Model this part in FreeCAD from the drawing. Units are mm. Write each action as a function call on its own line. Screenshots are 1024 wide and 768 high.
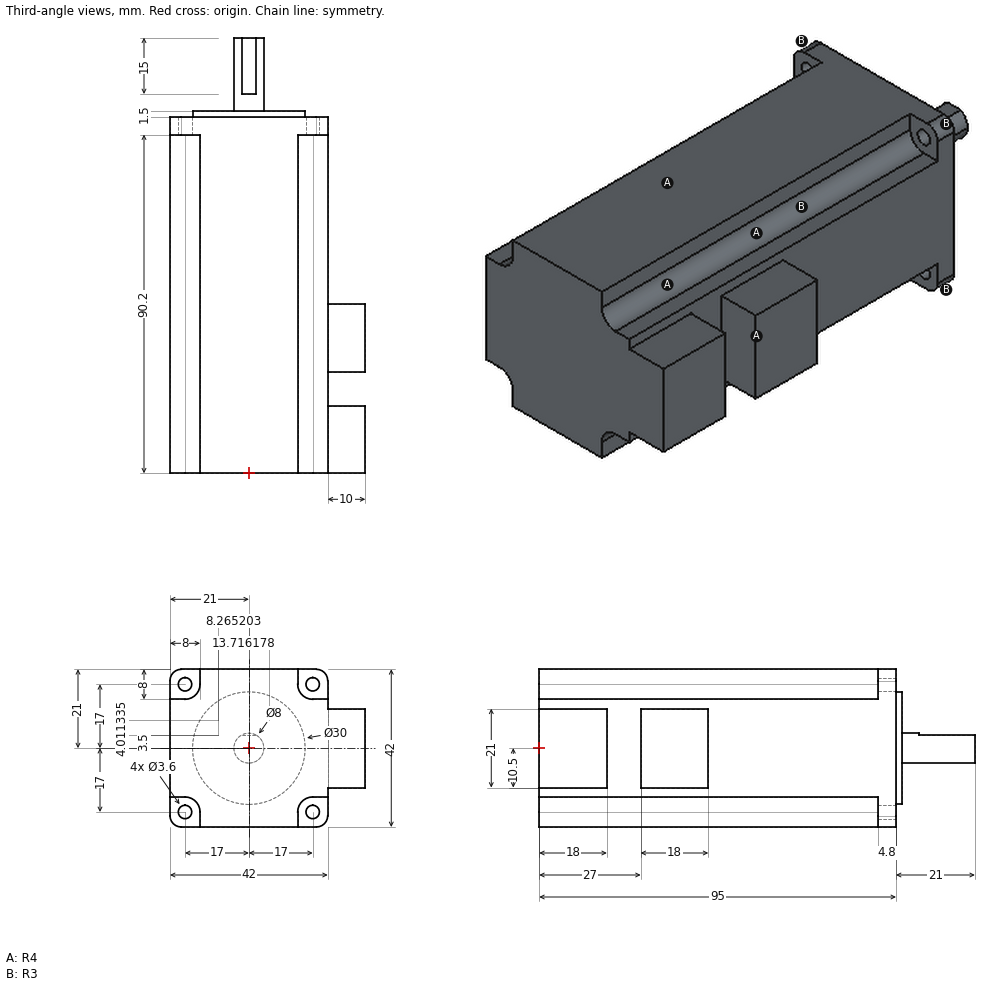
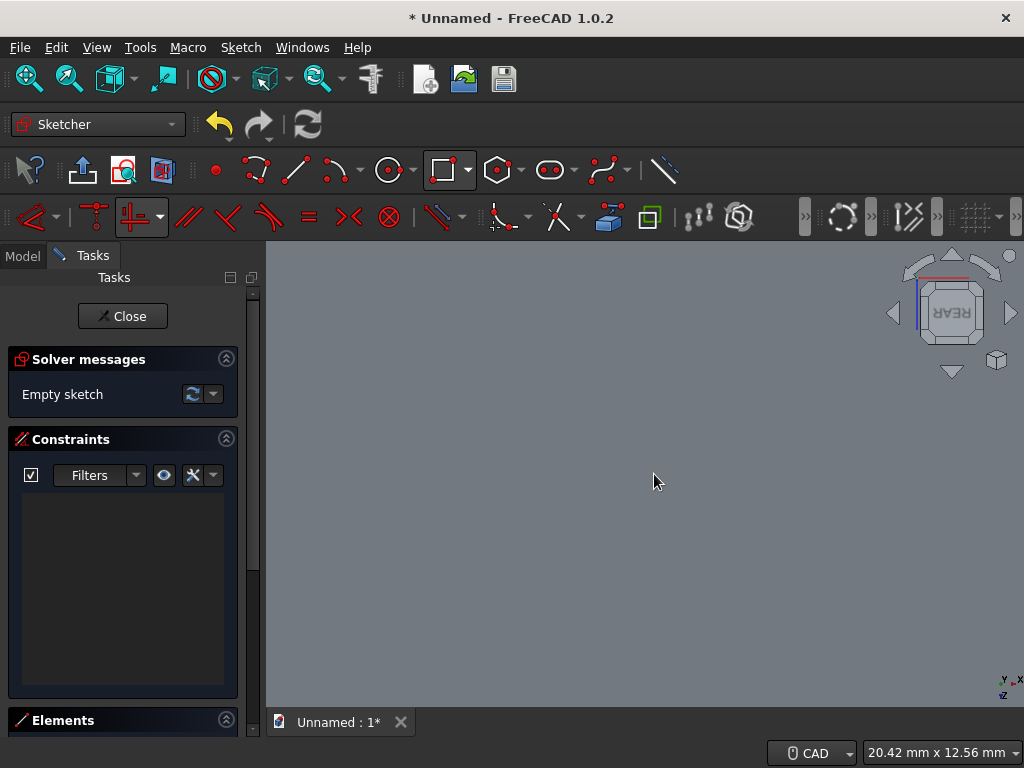
click(390, 170)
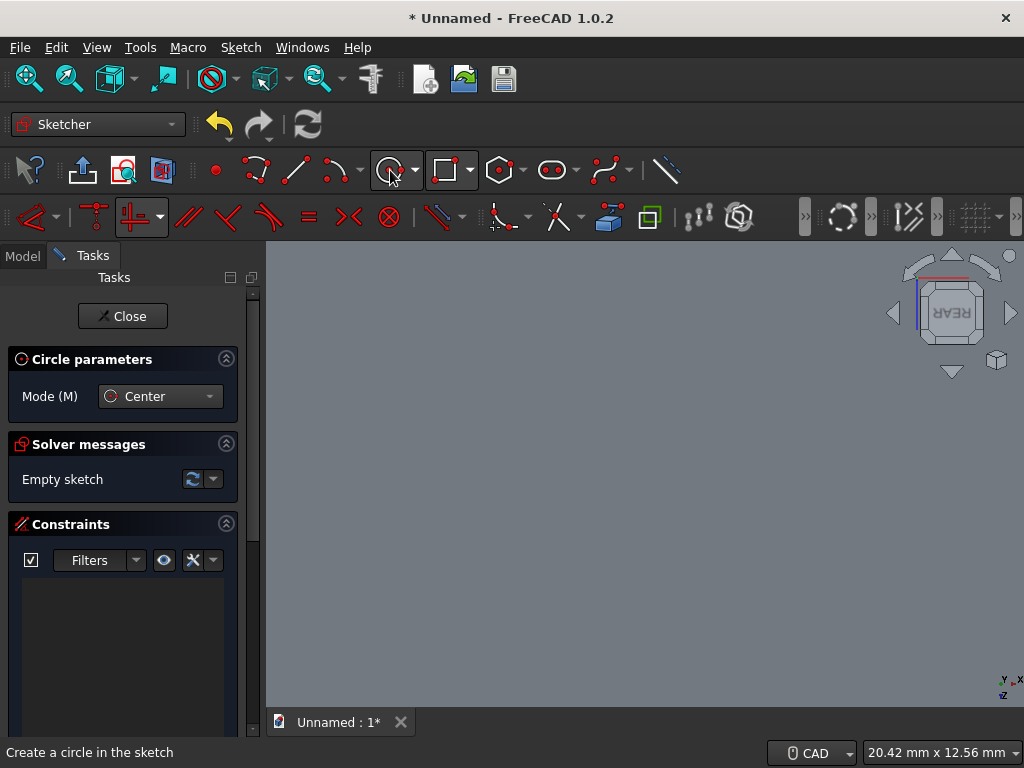
click(569, 470)
click(674, 365)
key(Escape)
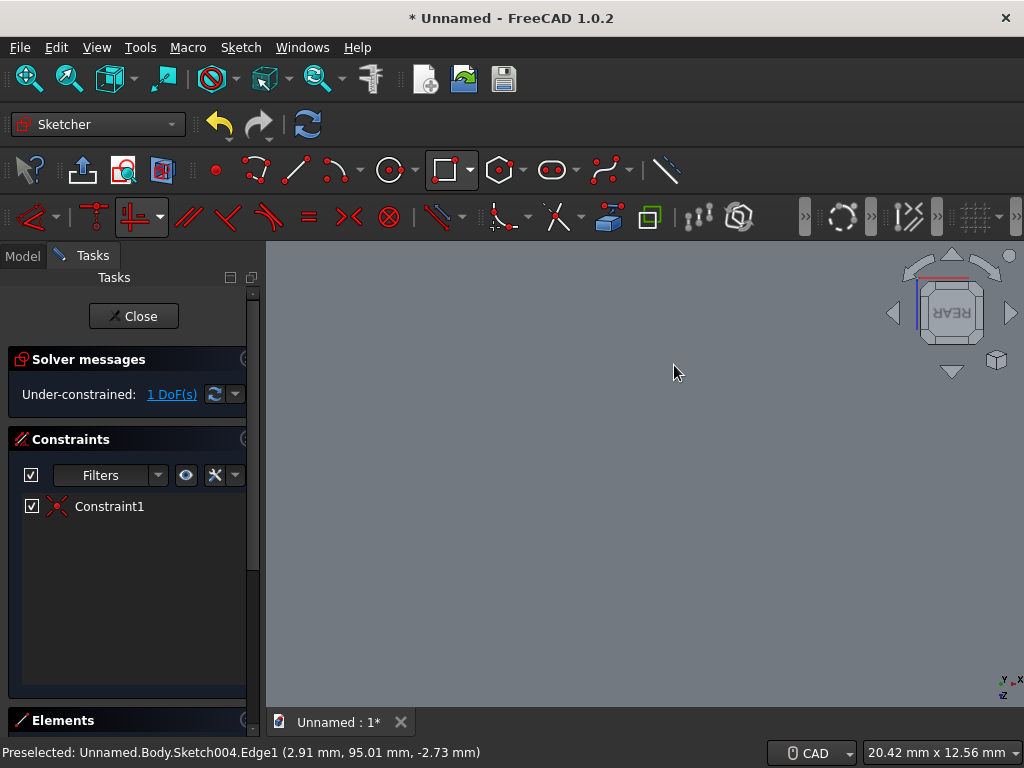
click(32, 218)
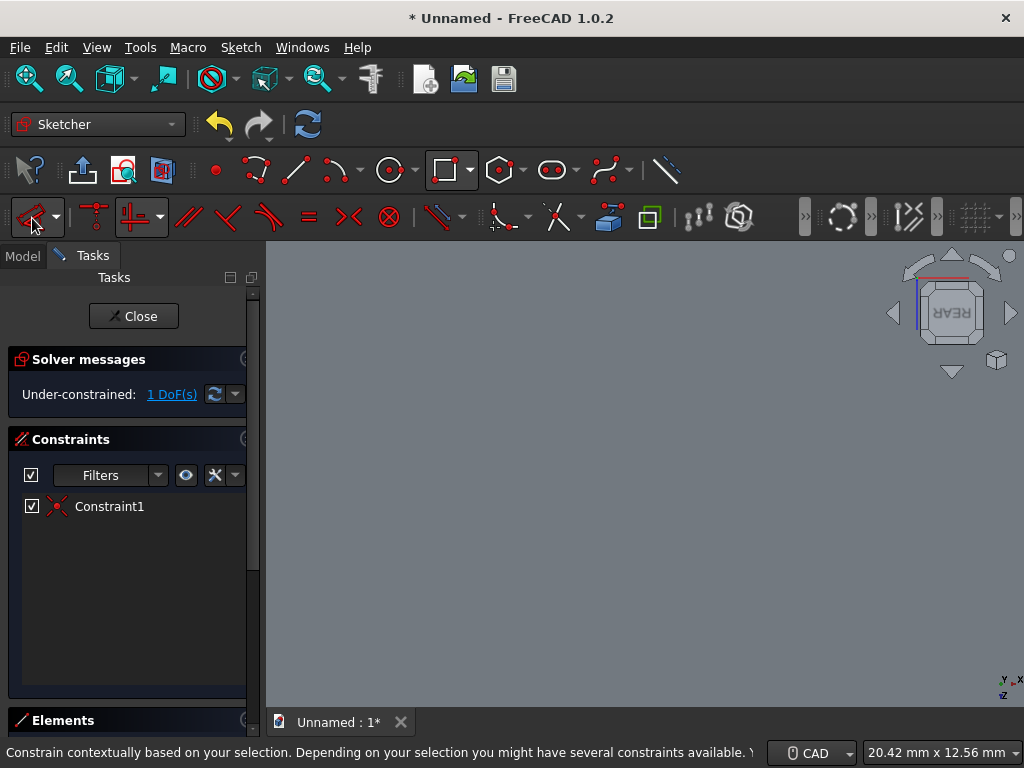
click(673, 365)
click(696, 342)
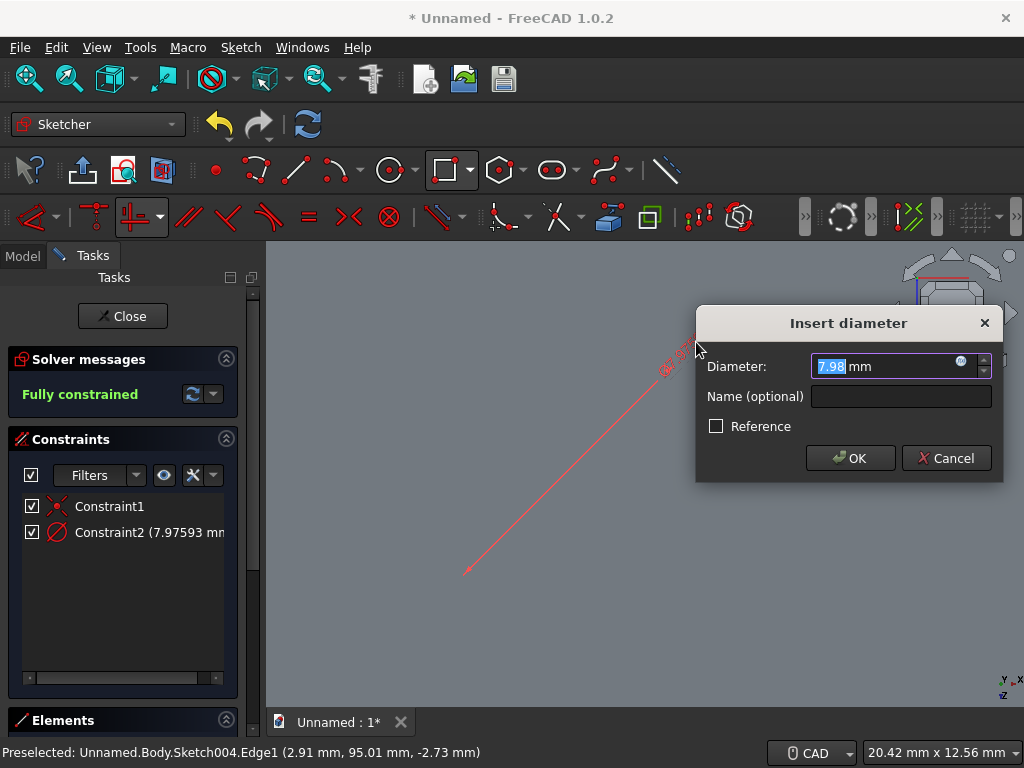
text(8)
key(Return)
key(Escape)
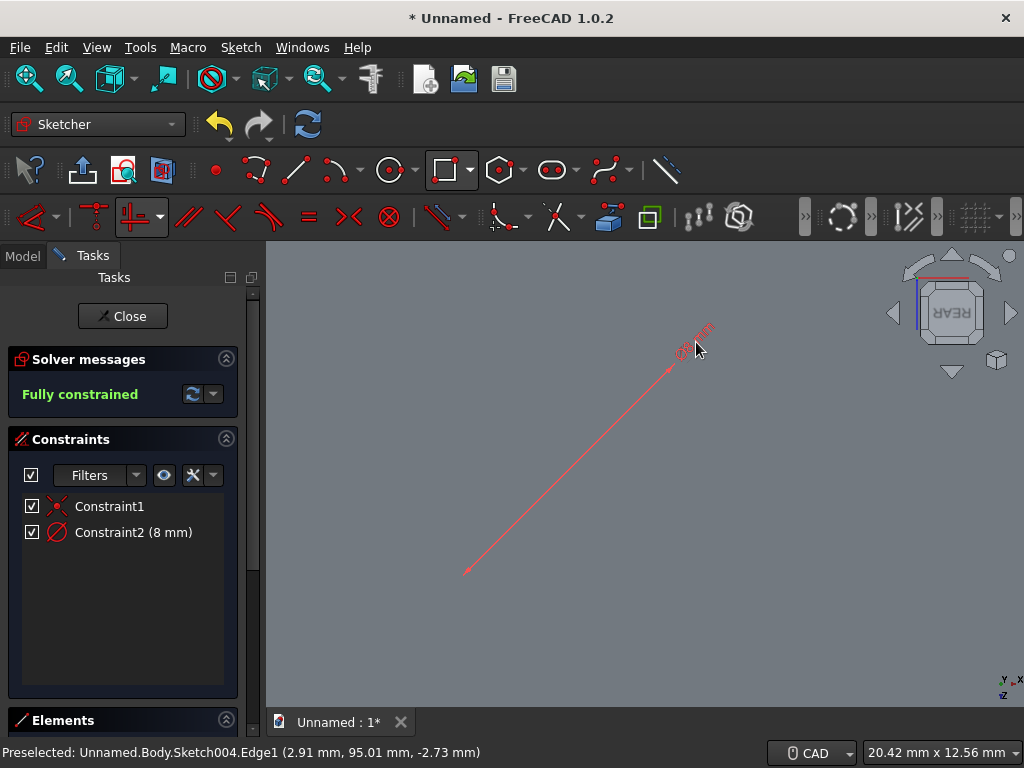
click(123, 316)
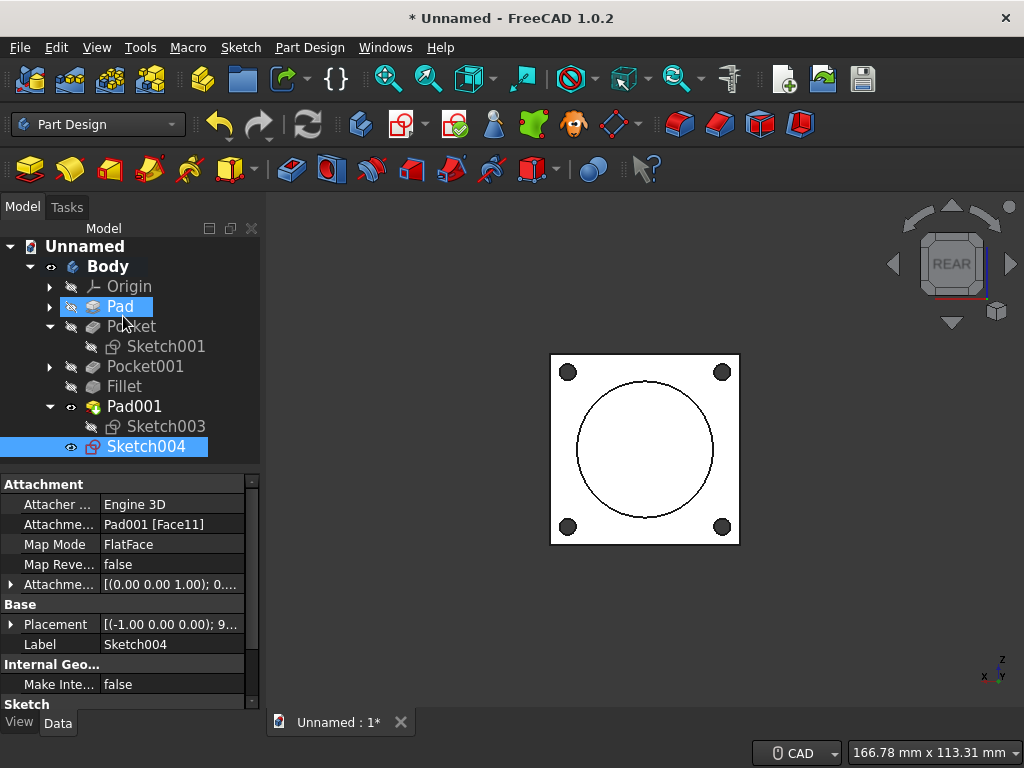
click(30, 170)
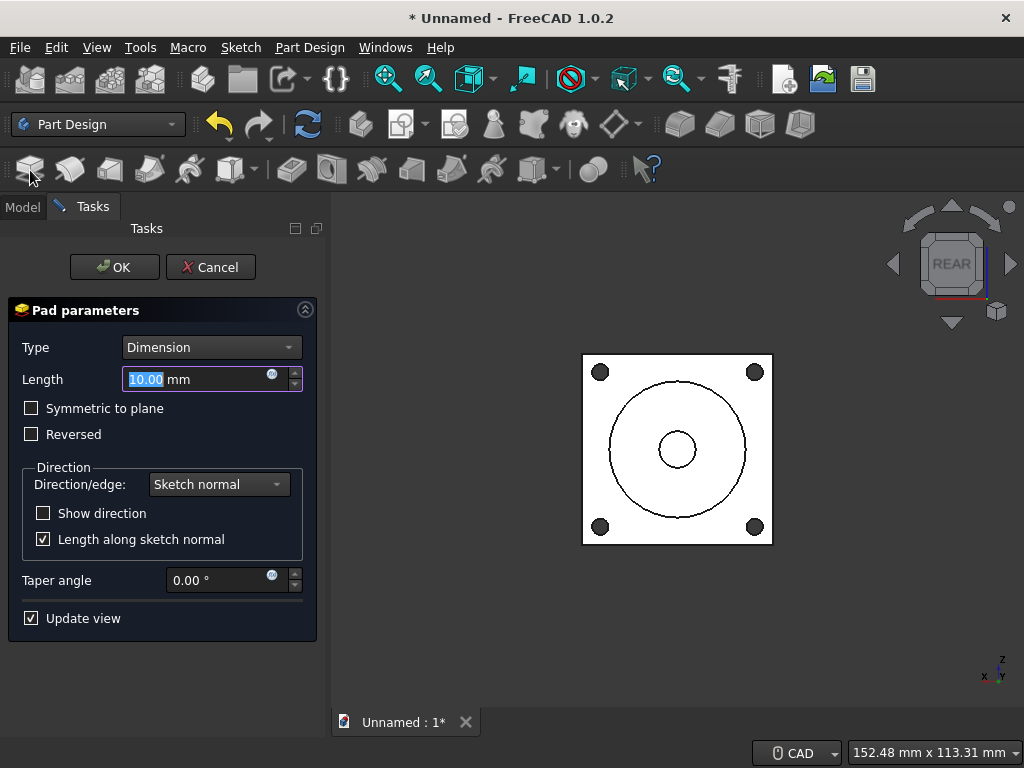
text(21)
key(Tab)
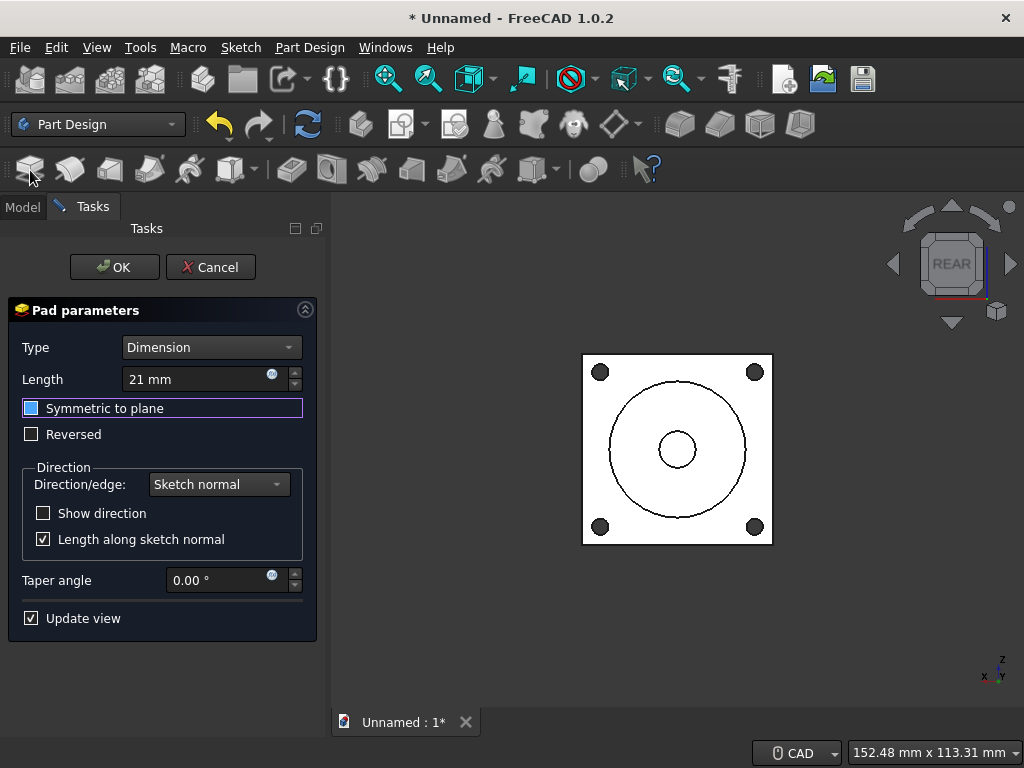
click(115, 267)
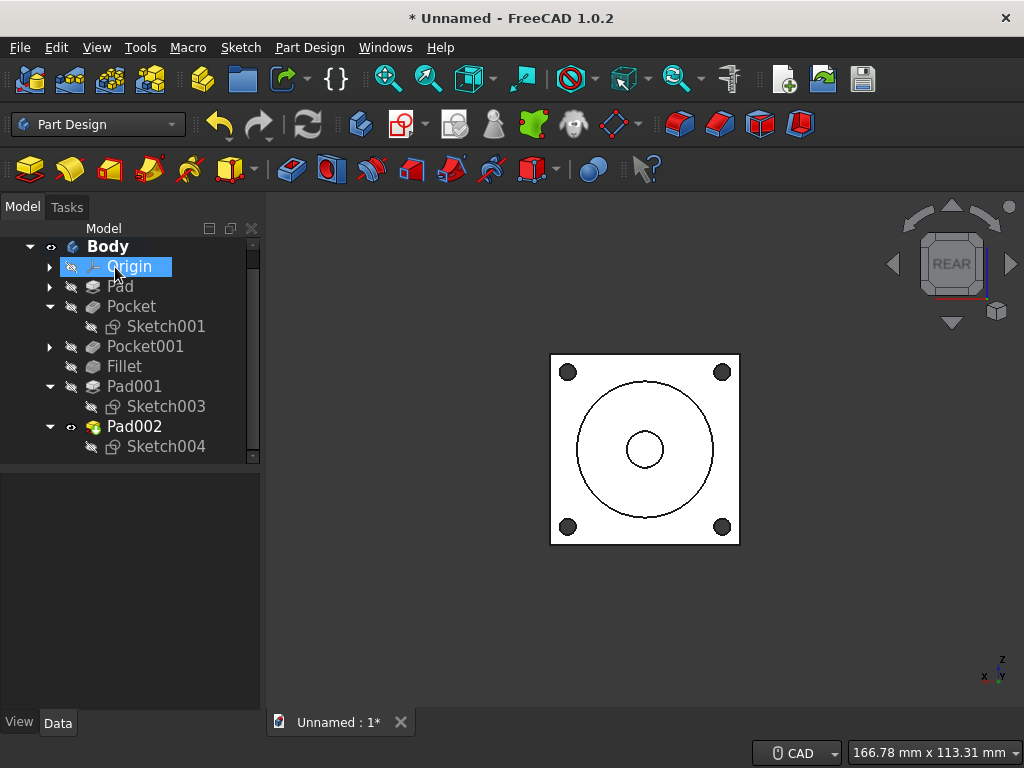
click(390, 80)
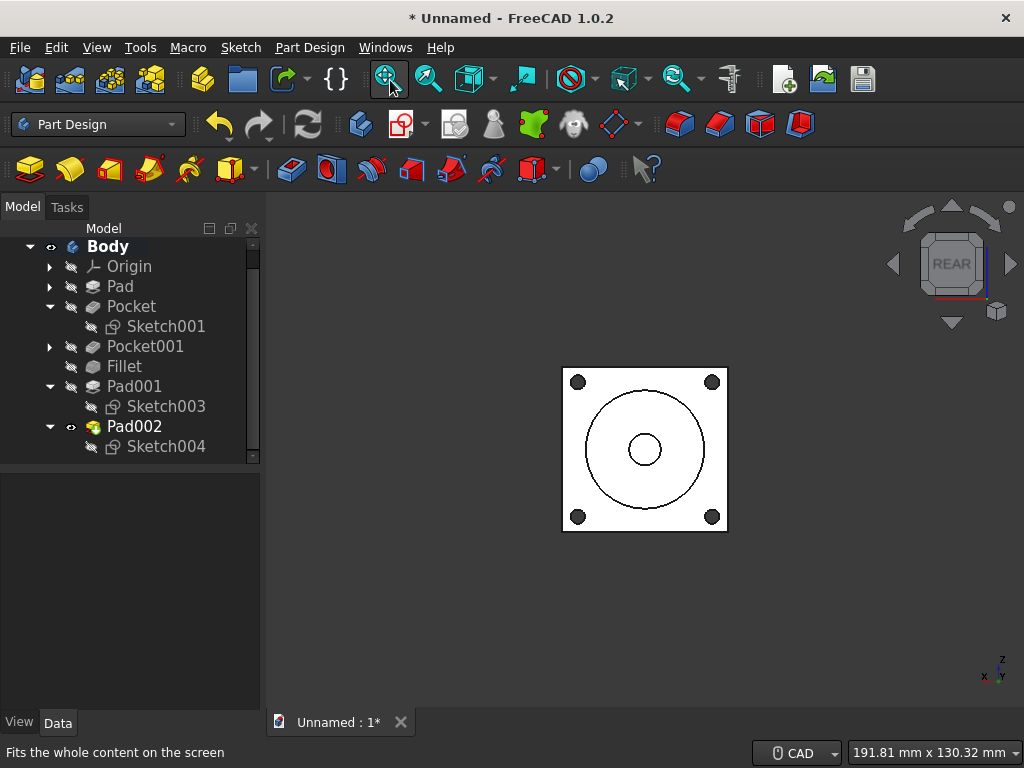
scroll(562, 366, up, 4)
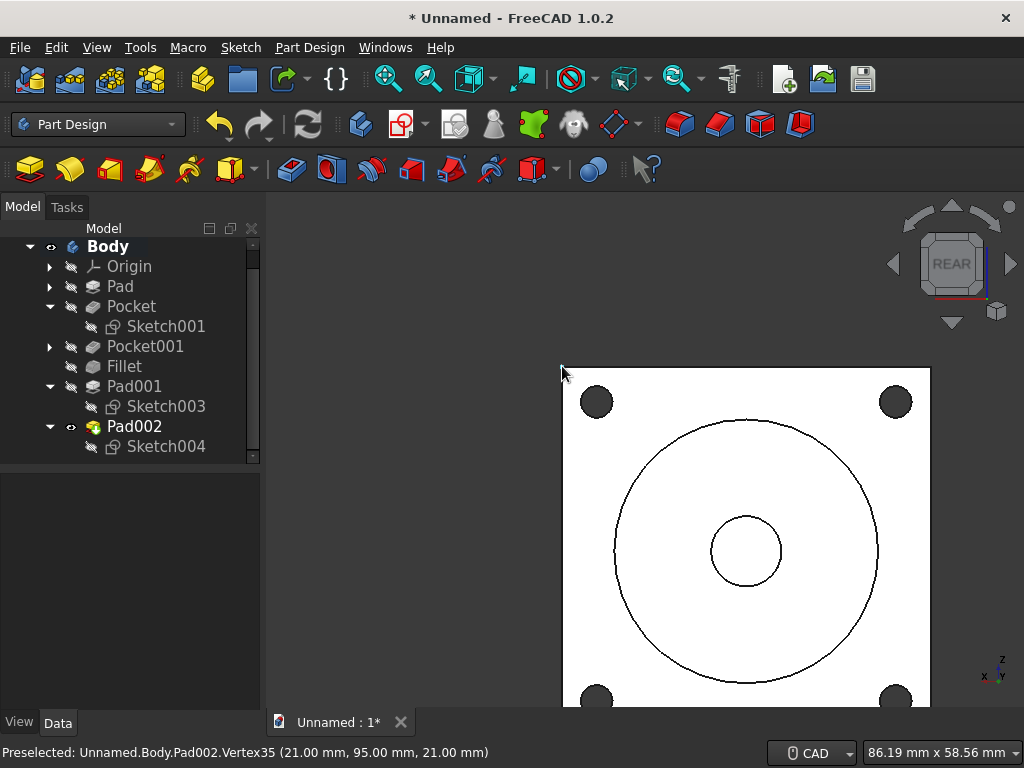
click(390, 80)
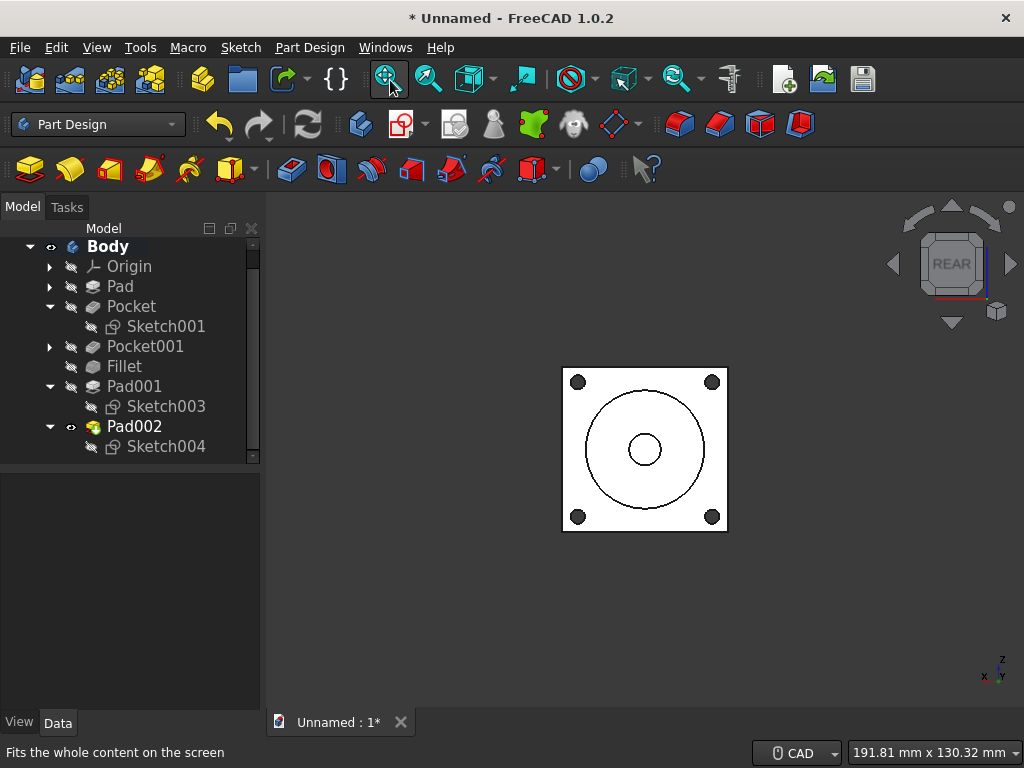
key(0)